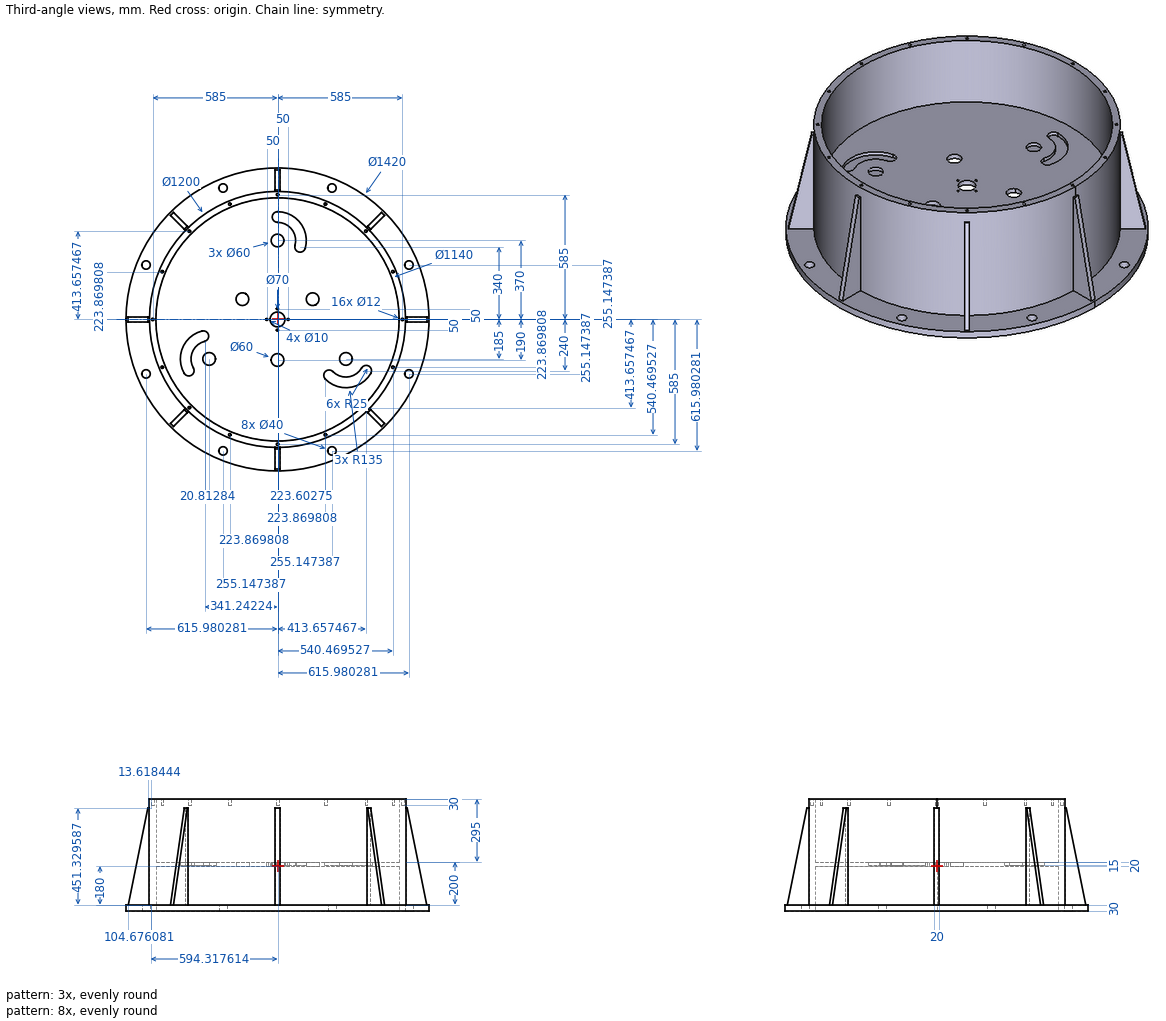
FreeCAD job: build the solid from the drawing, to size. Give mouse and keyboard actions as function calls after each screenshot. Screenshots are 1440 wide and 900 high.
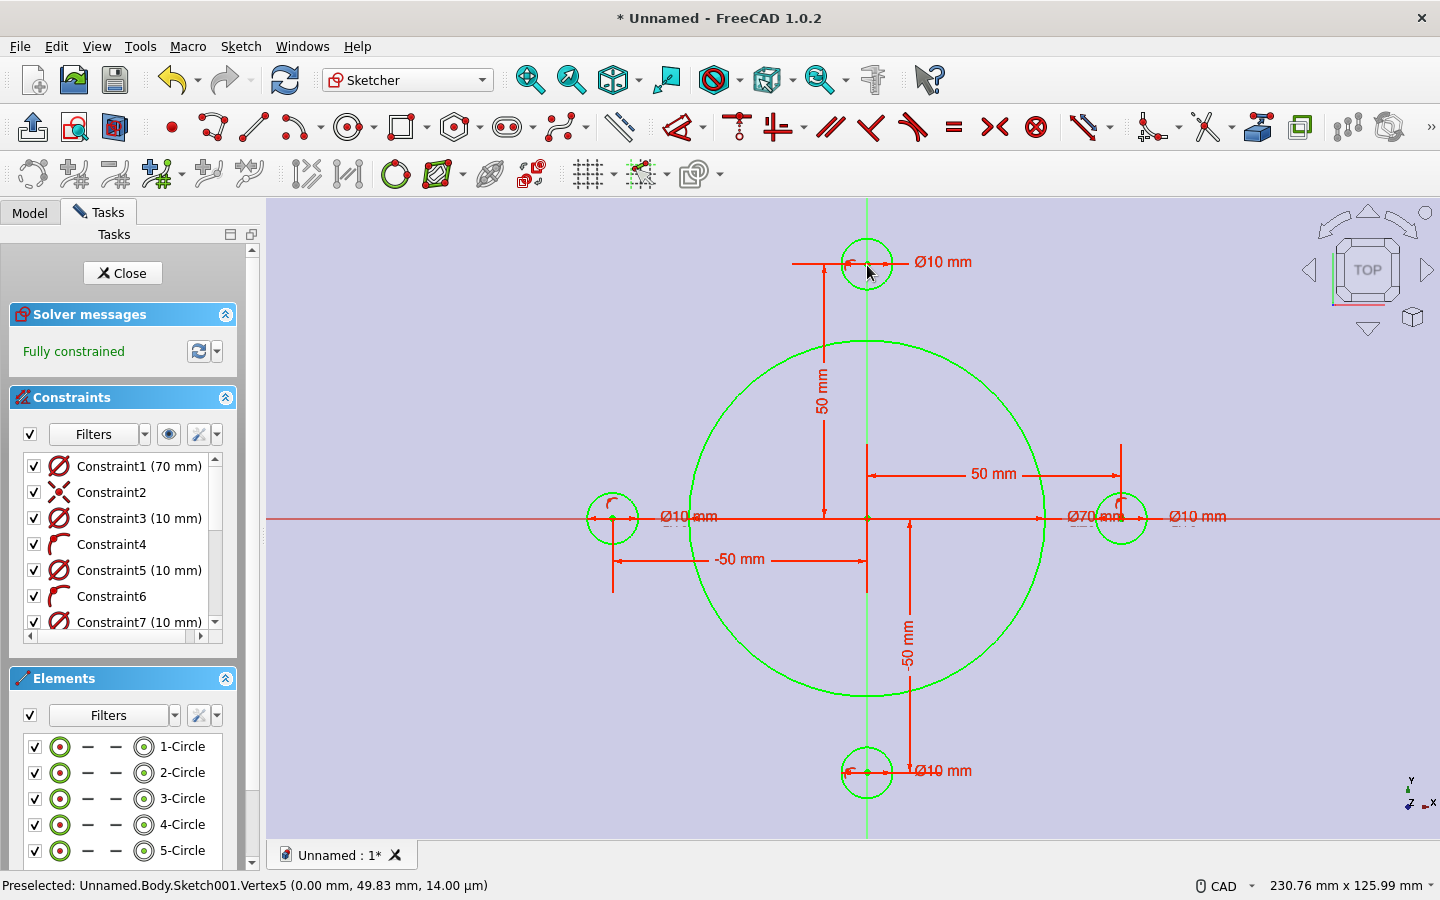
click(123, 273)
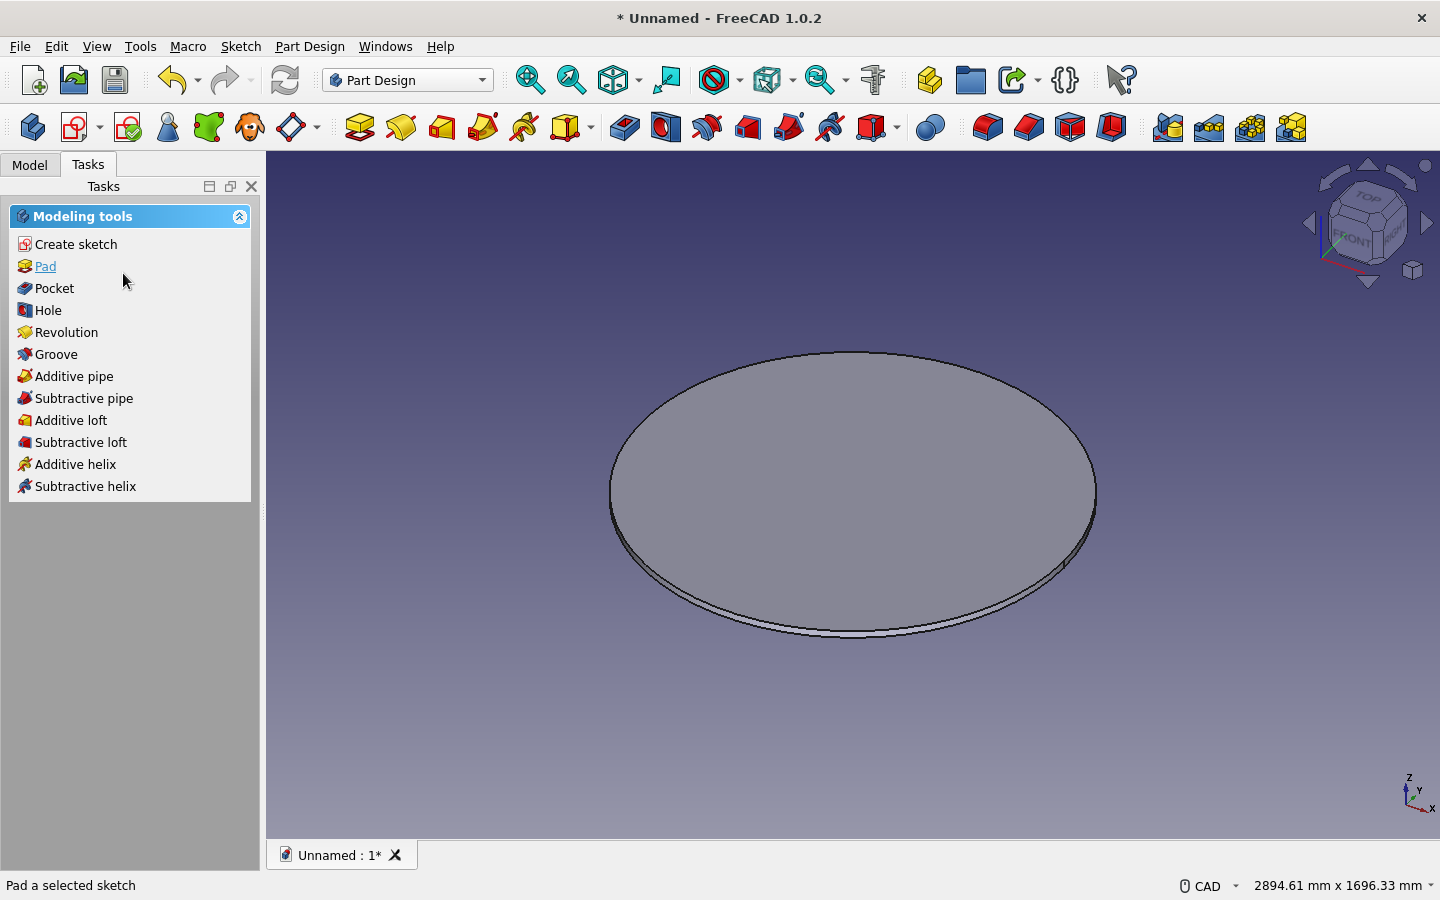
click(625, 128)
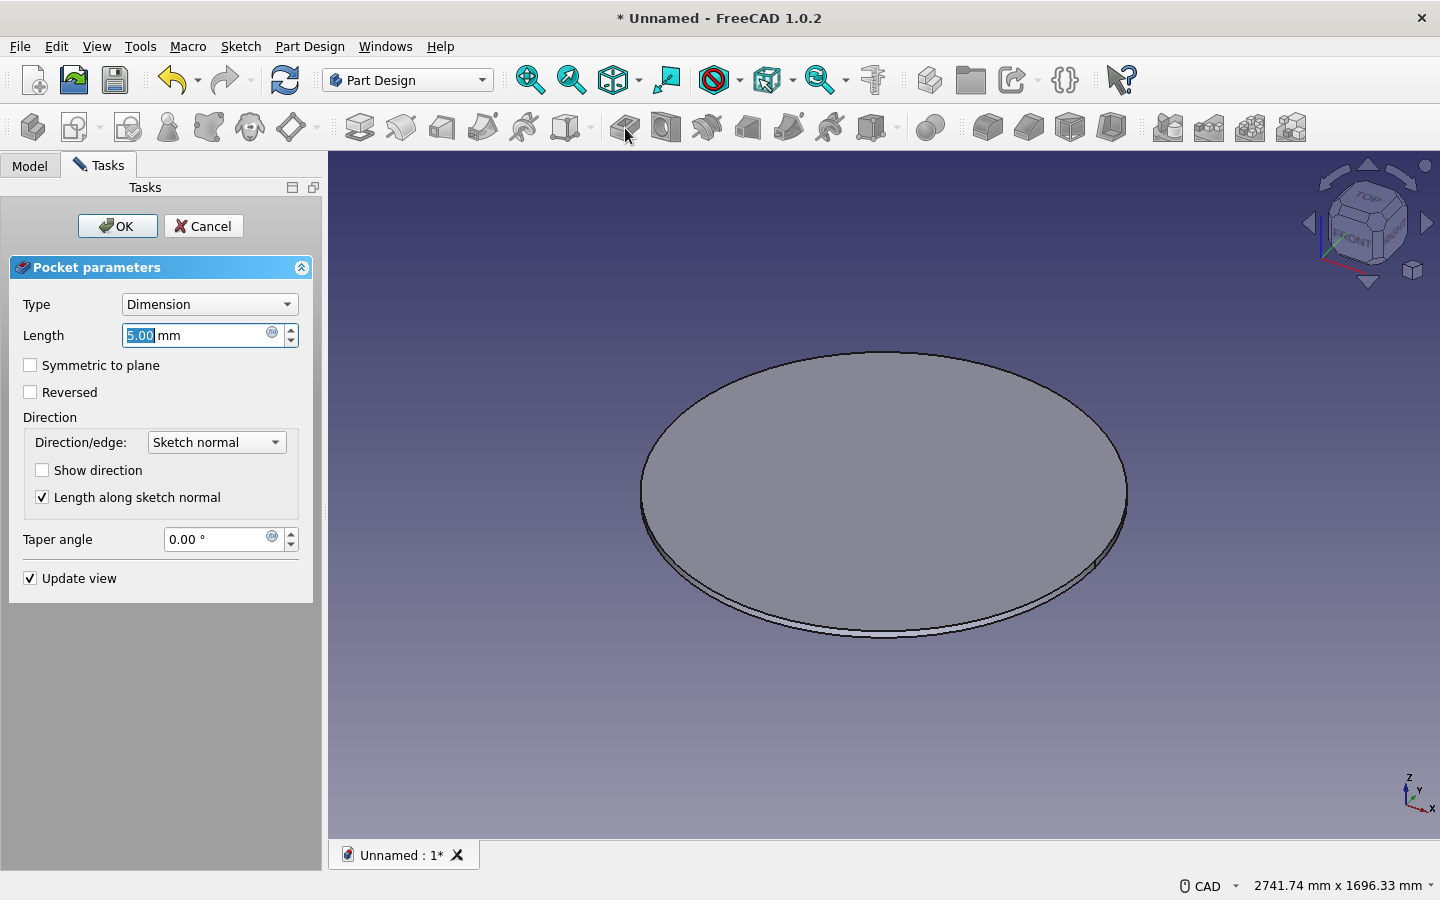
click(210, 304)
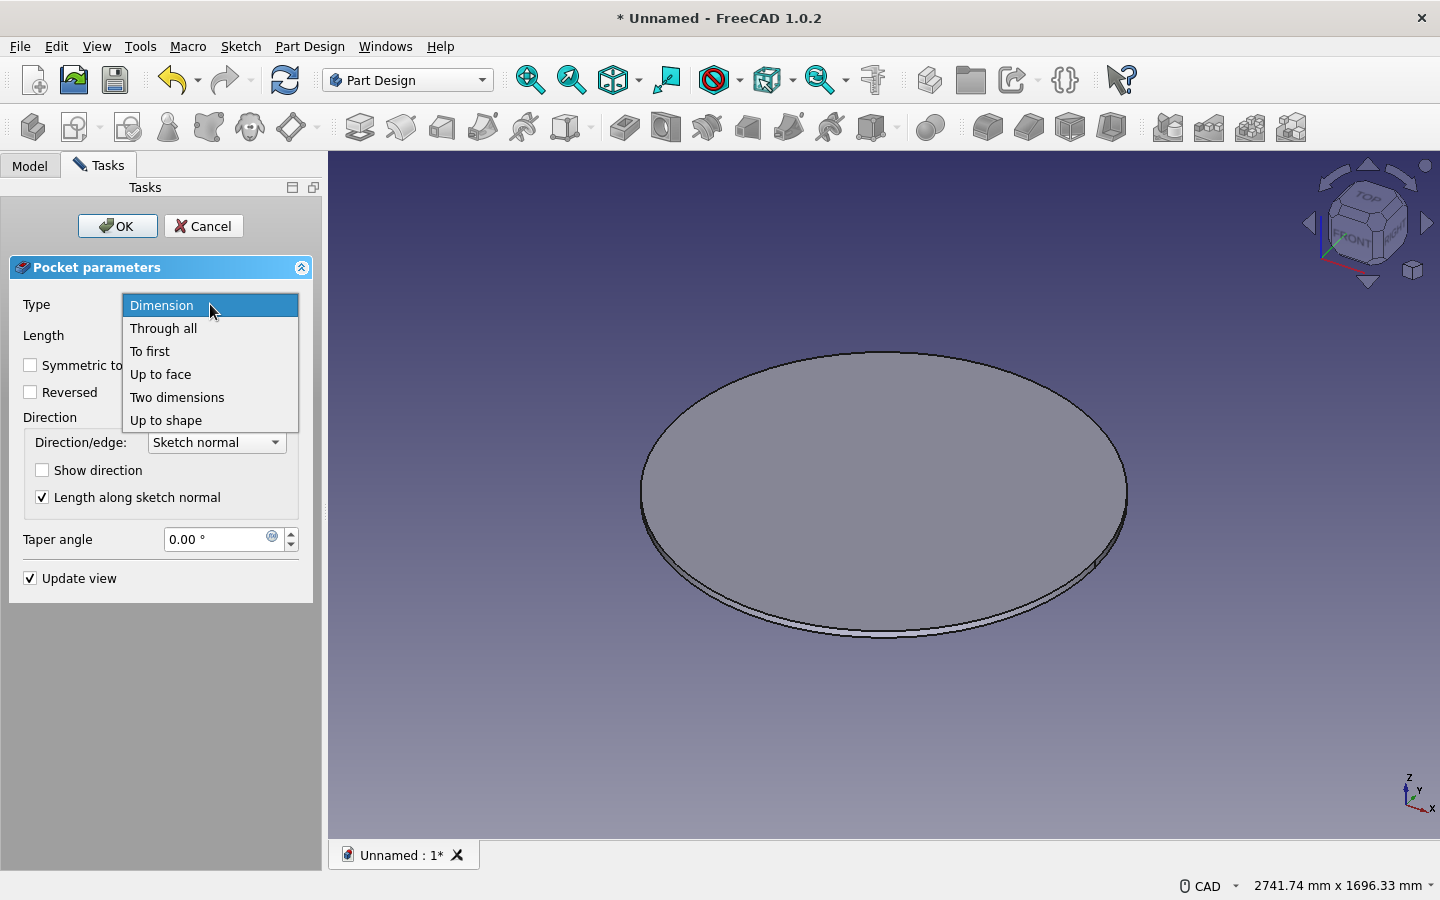
click(208, 328)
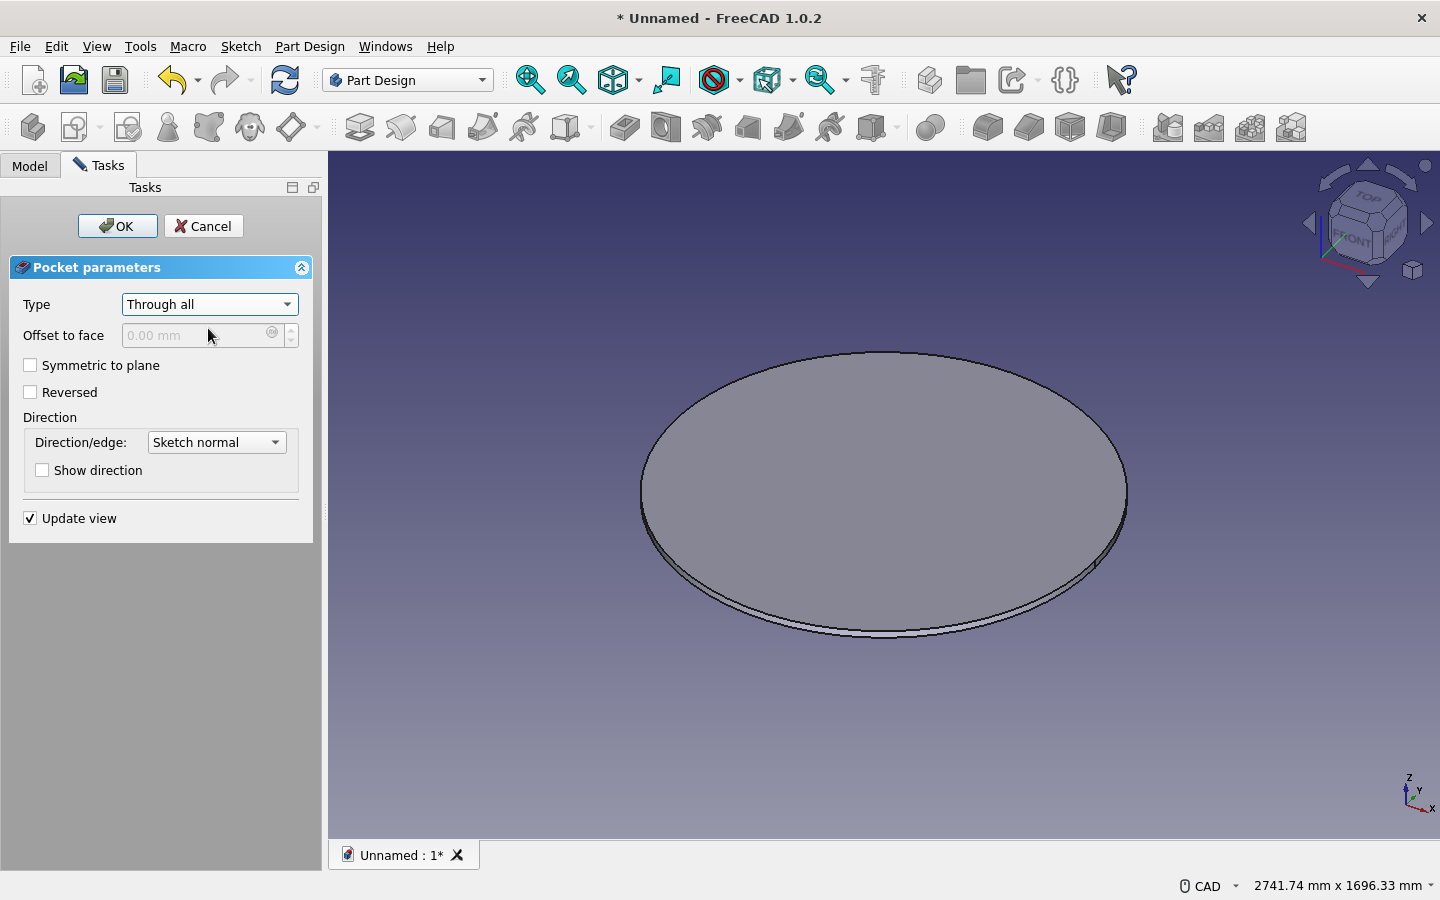
click(31, 392)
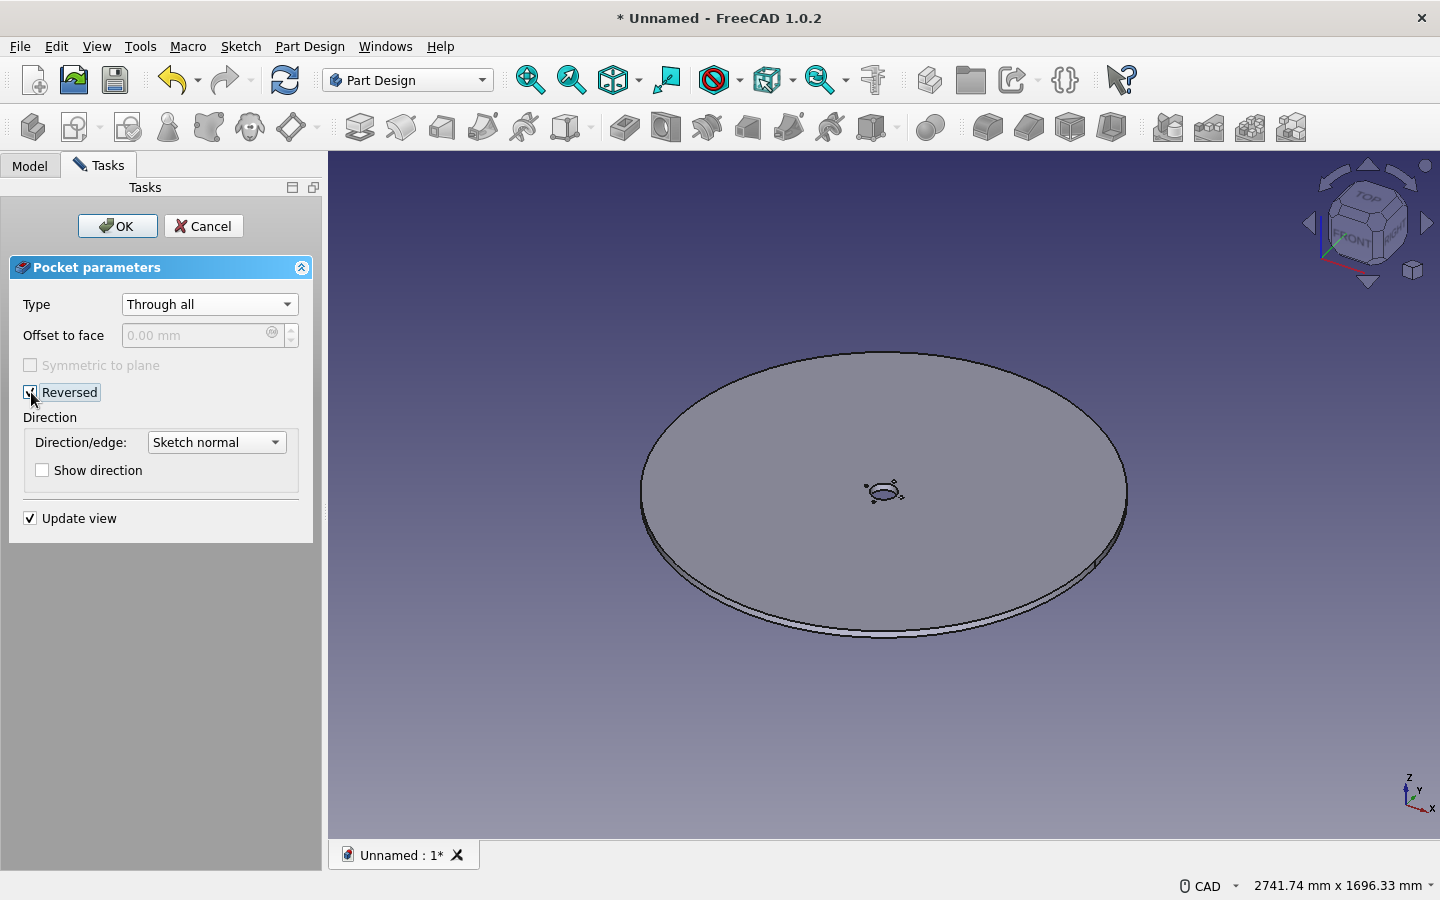
click(118, 226)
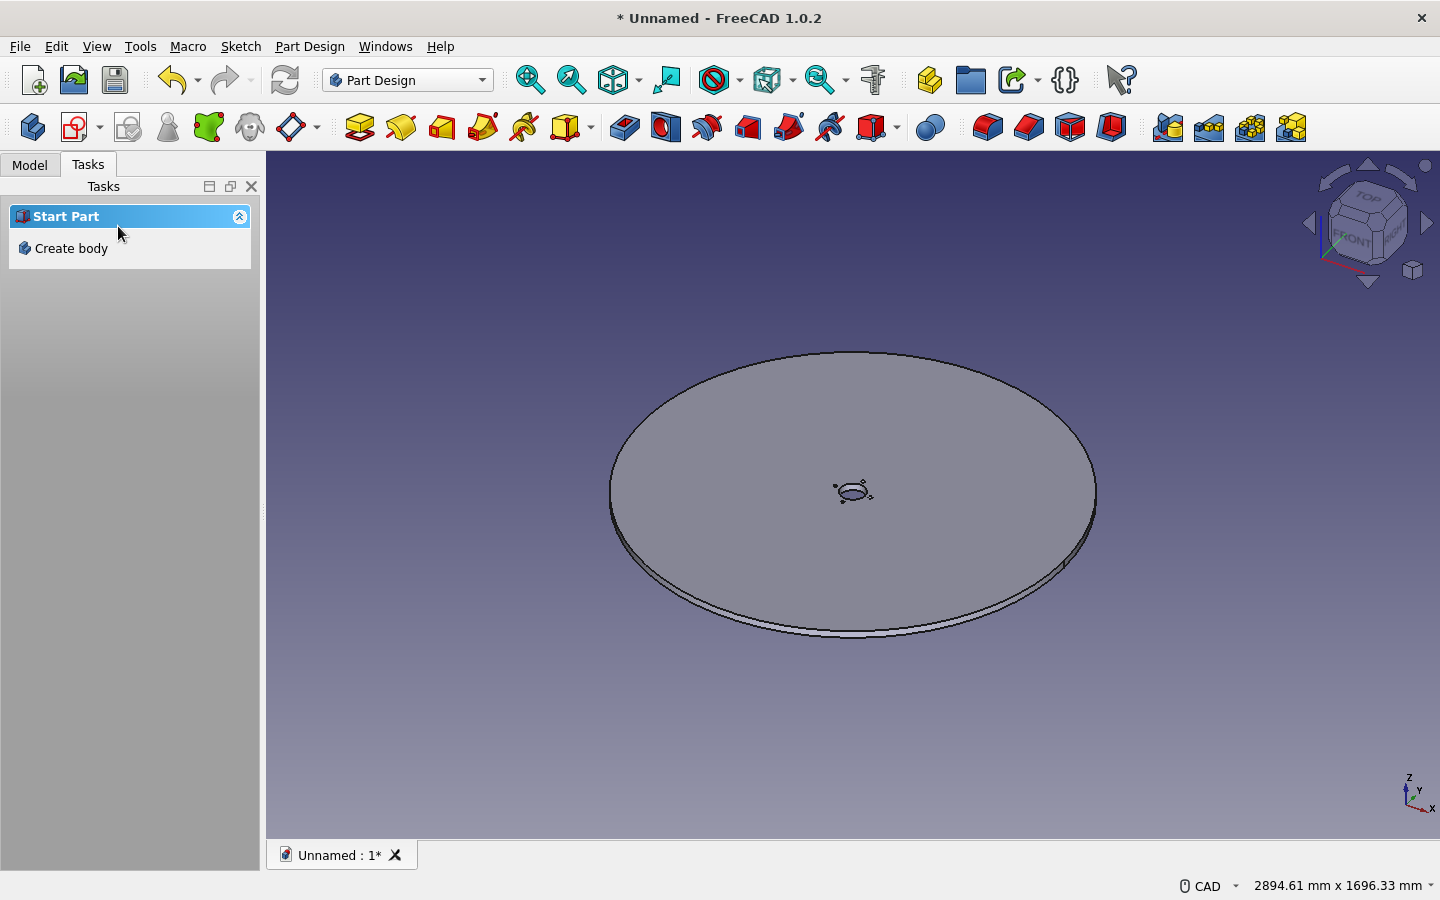
key(5)